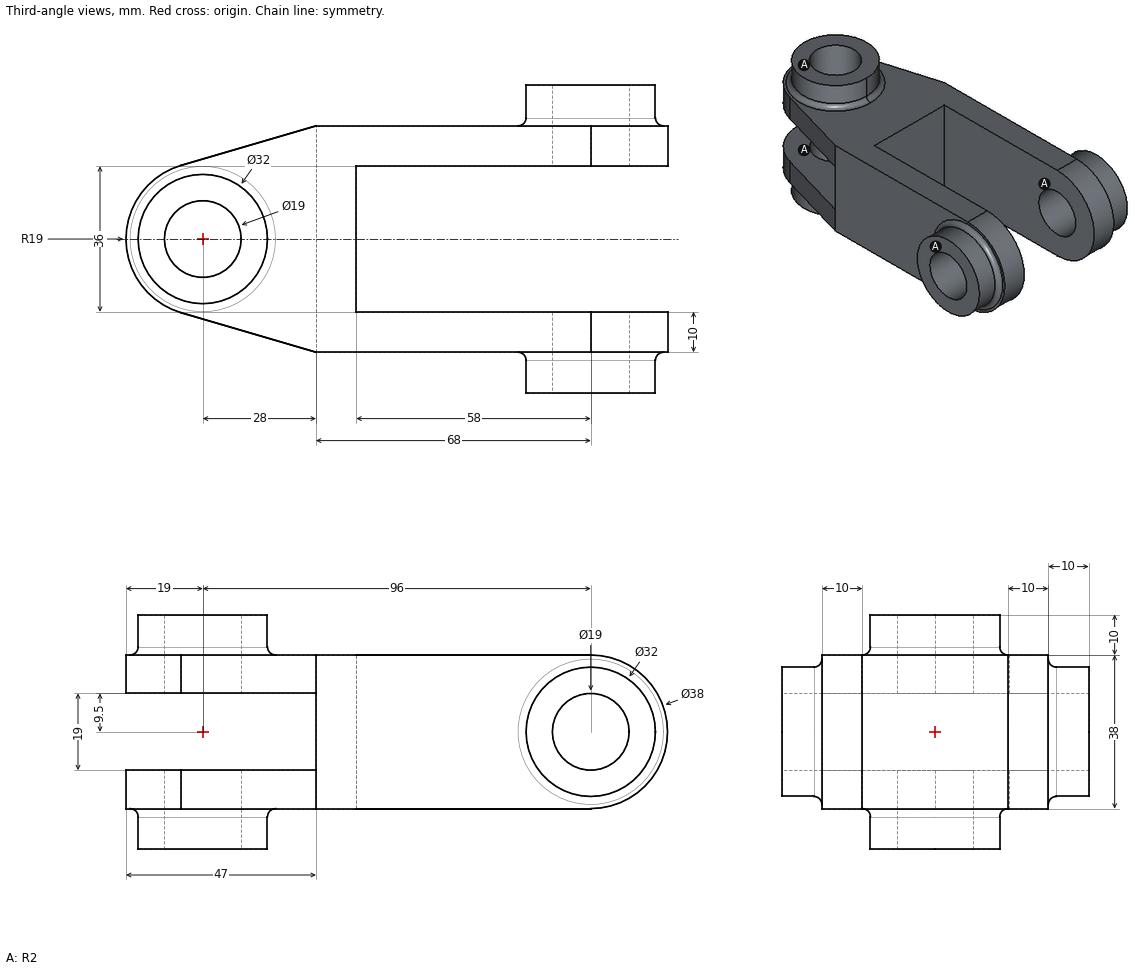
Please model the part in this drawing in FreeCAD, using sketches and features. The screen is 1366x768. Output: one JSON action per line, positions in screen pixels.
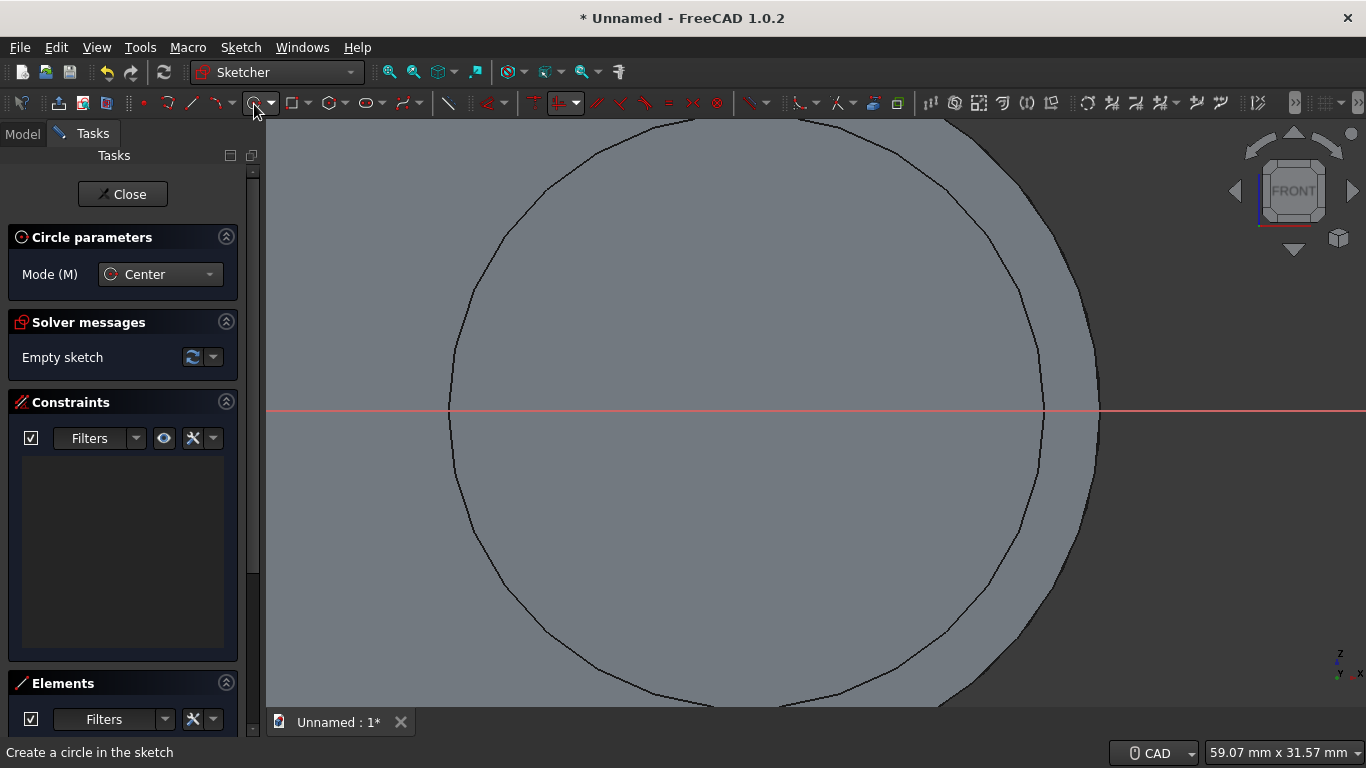
{"action": "left_click", "coordinate": [746, 411]}
{"action": "left_click", "coordinate": [872, 286]}
{"action": "key", "text": "Escape"}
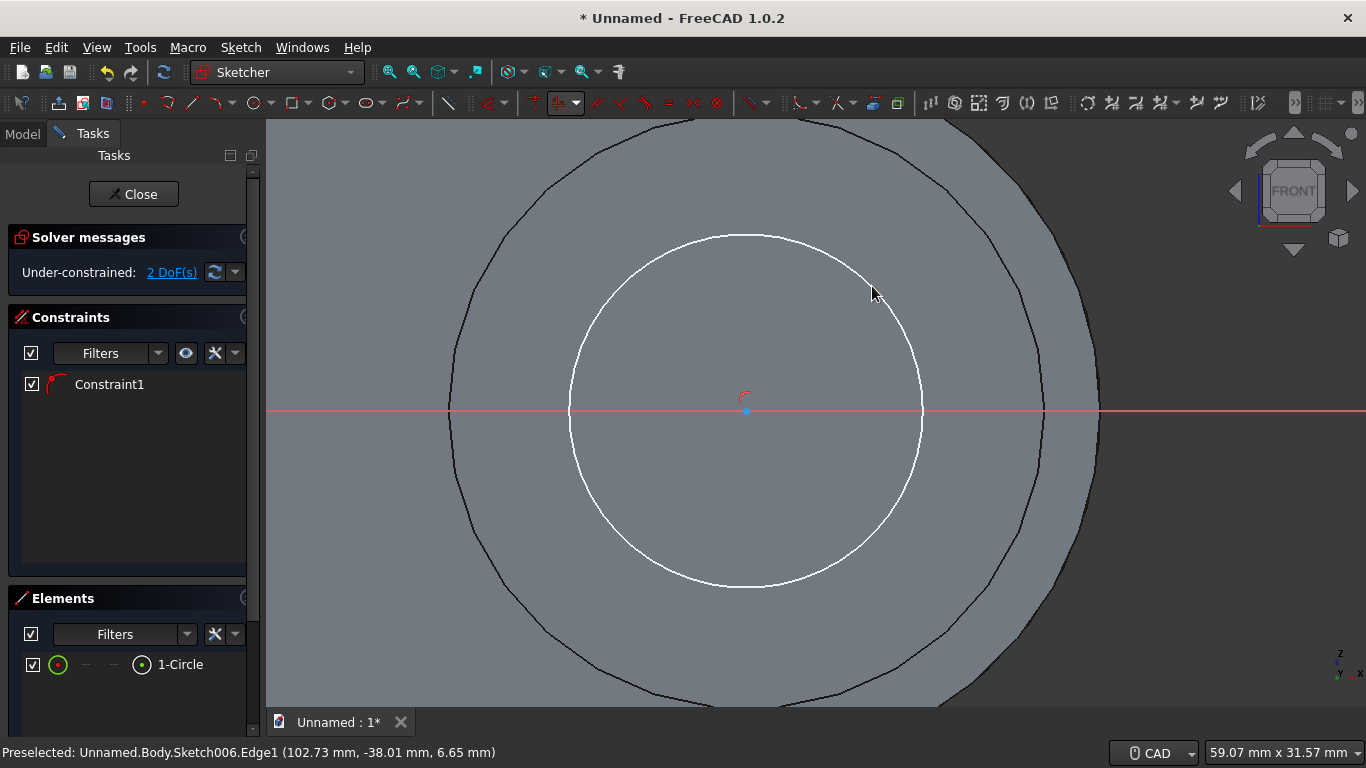
{"action": "left_click", "coordinate": [488, 104]}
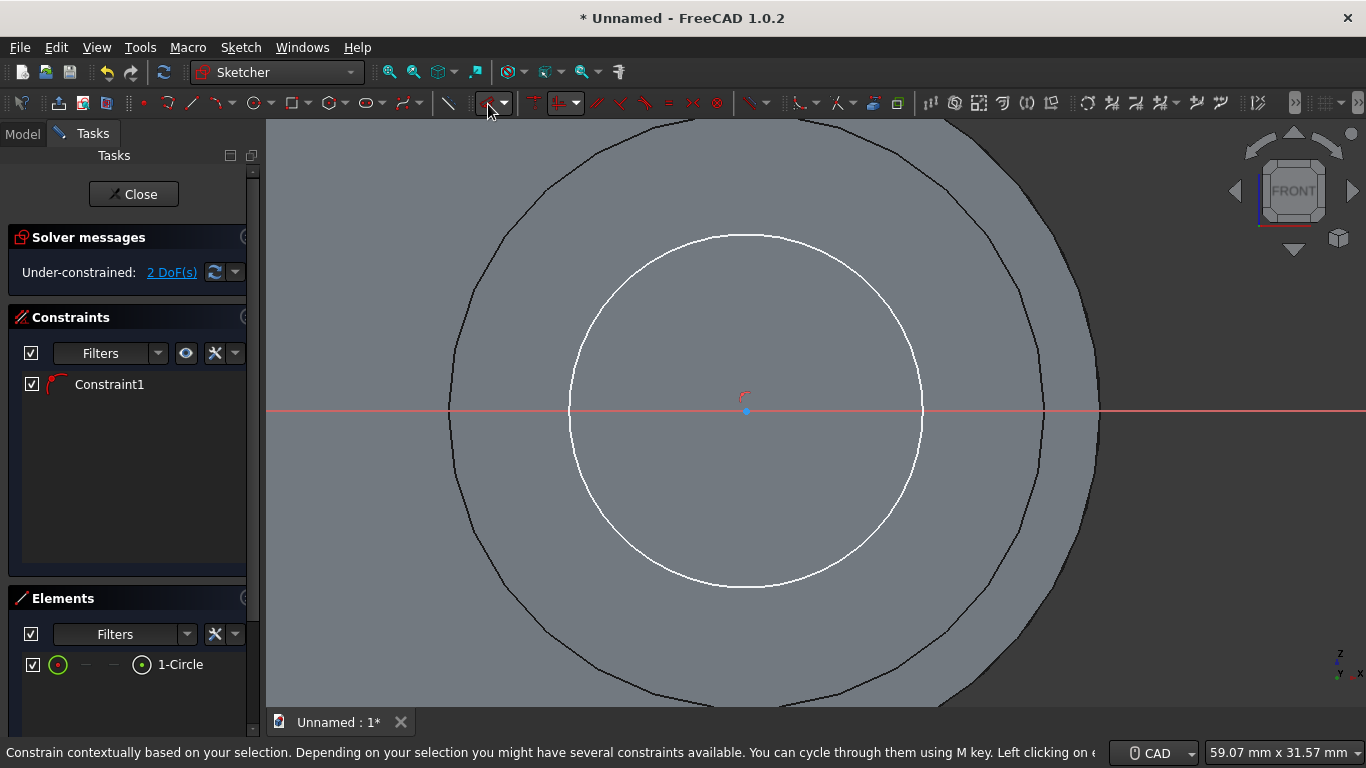
{"action": "left_click", "coordinate": [871, 286]}
{"action": "left_click", "coordinate": [894, 263]}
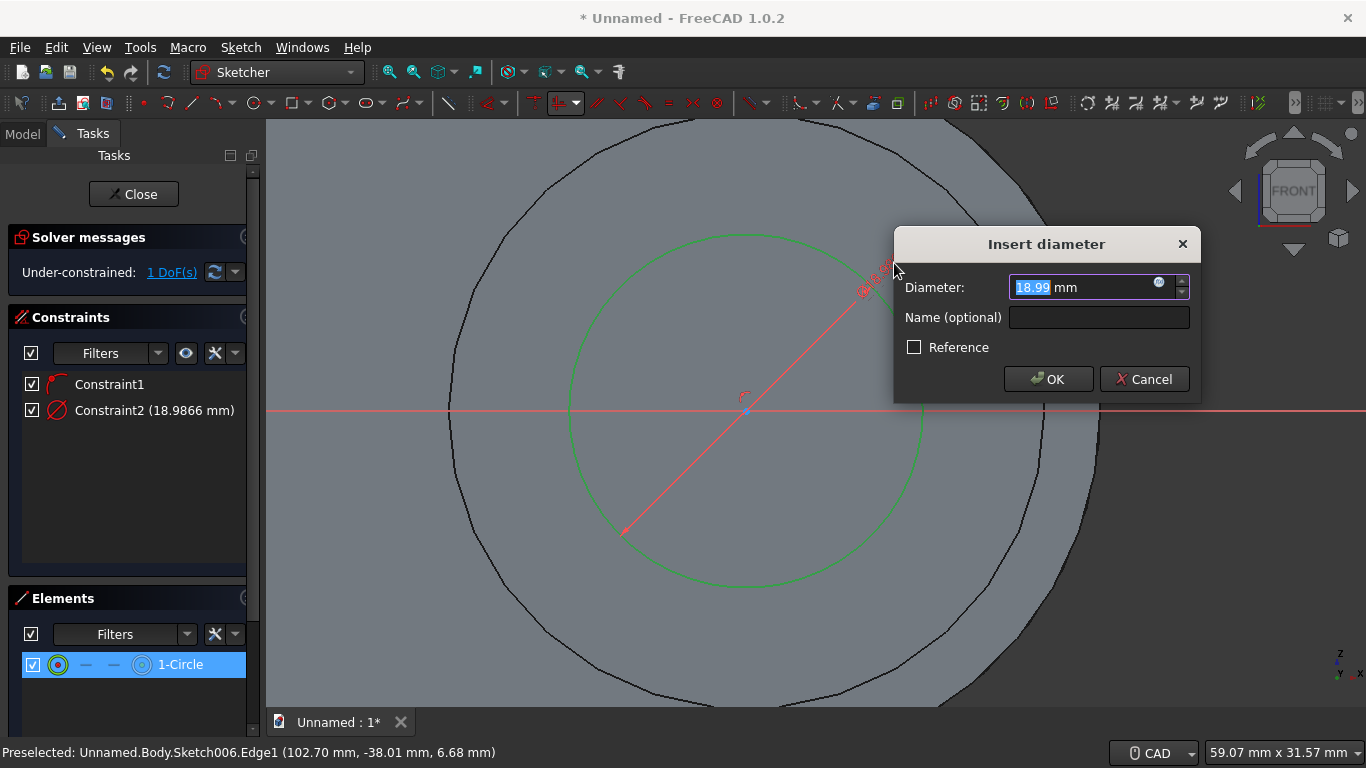
{"action": "type", "text": "19"}
{"action": "key", "text": "Return"}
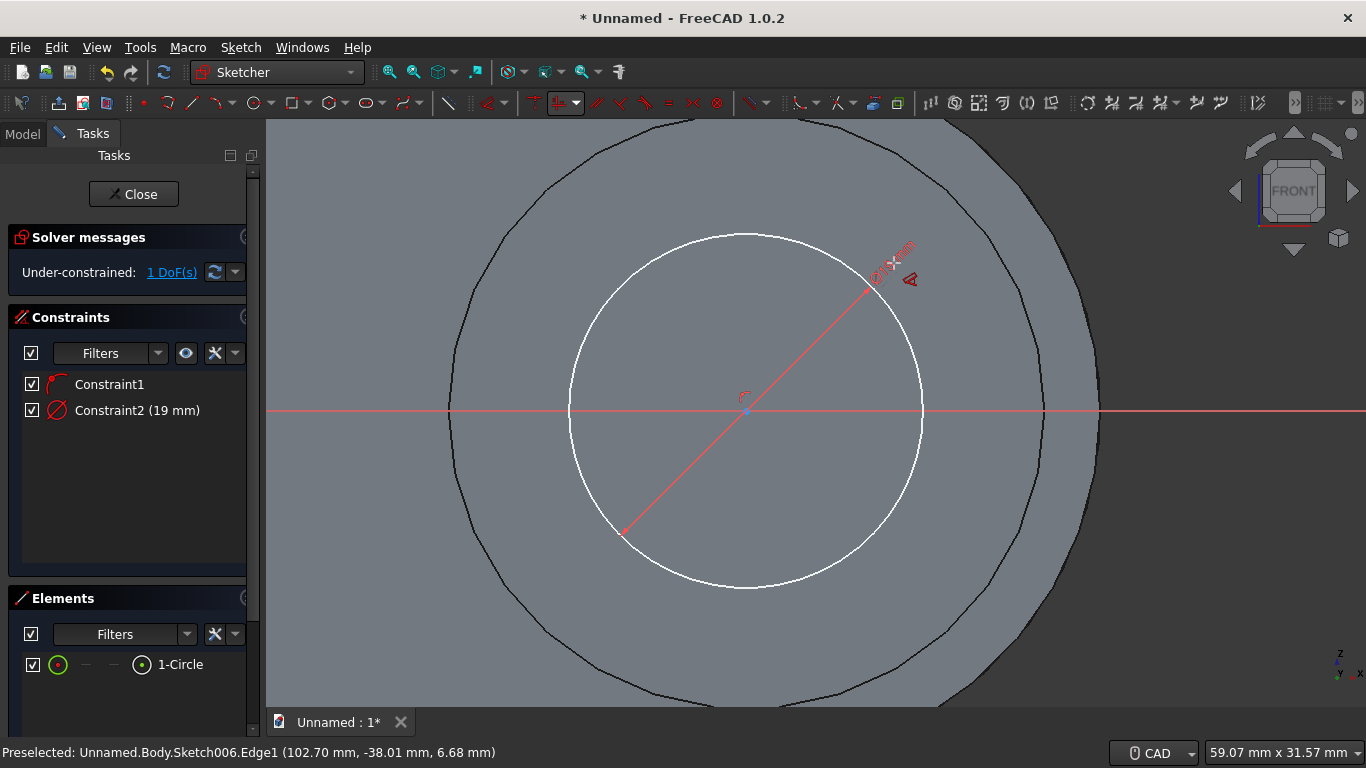
{"action": "left_click", "coordinate": [746, 411]}
{"action": "left_click", "coordinate": [520, 445]}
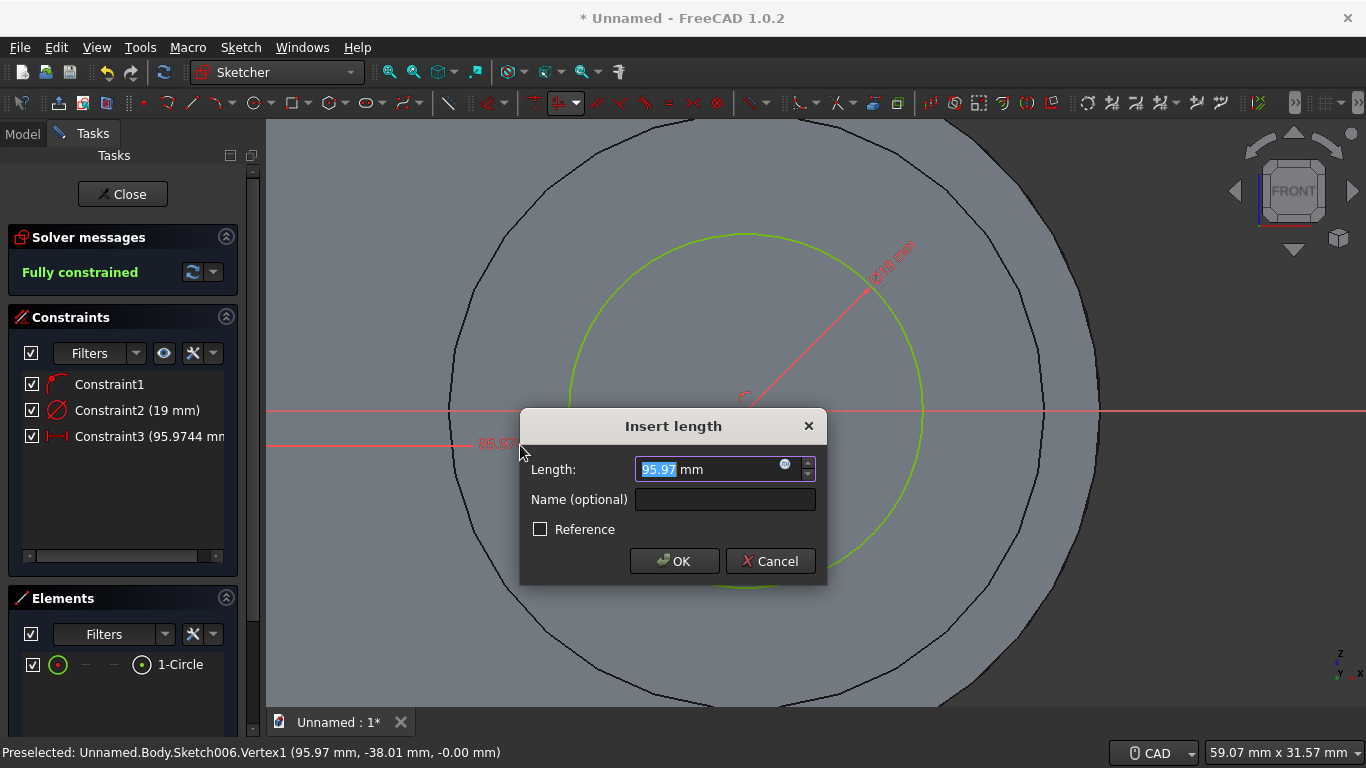
{"action": "type", "text": "96"}
{"action": "key", "text": "Return"}
{"action": "key", "text": "Escape"}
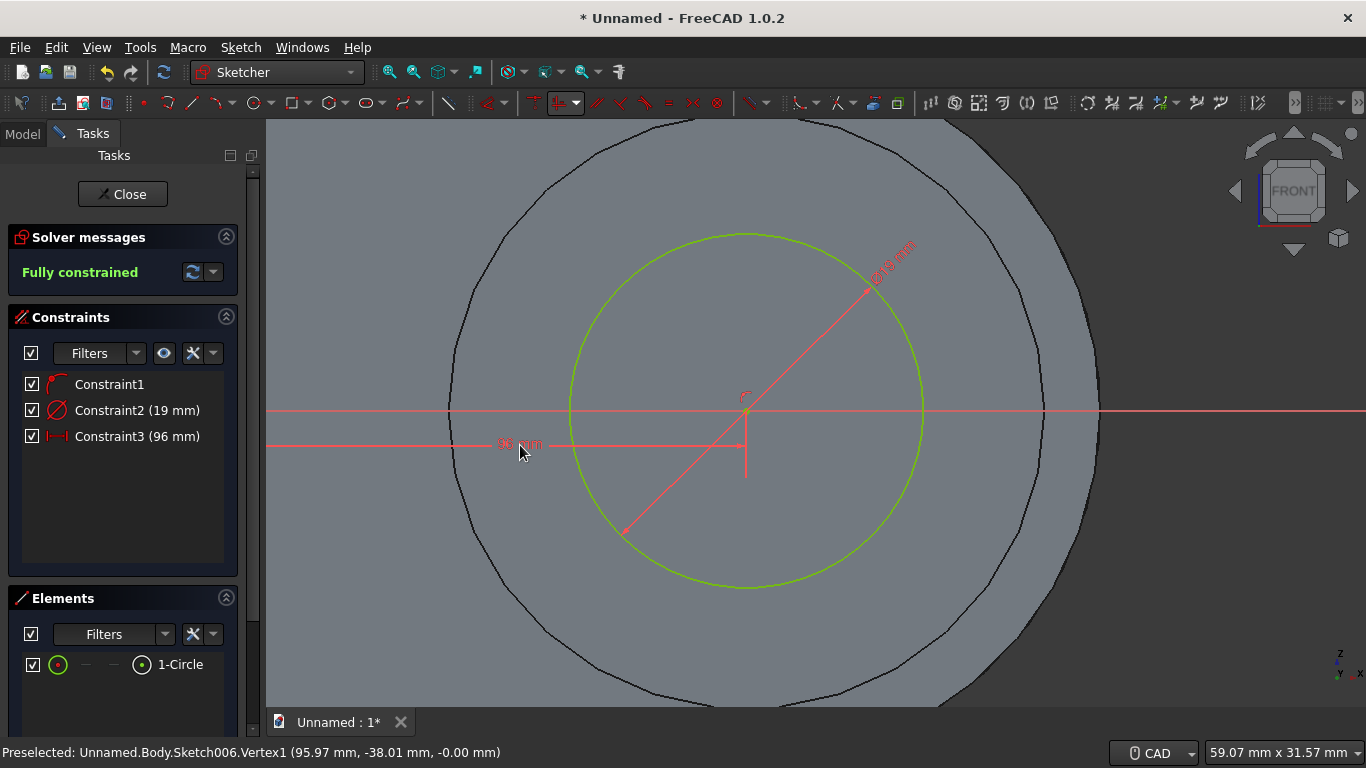
{"action": "left_click", "coordinate": [123, 194]}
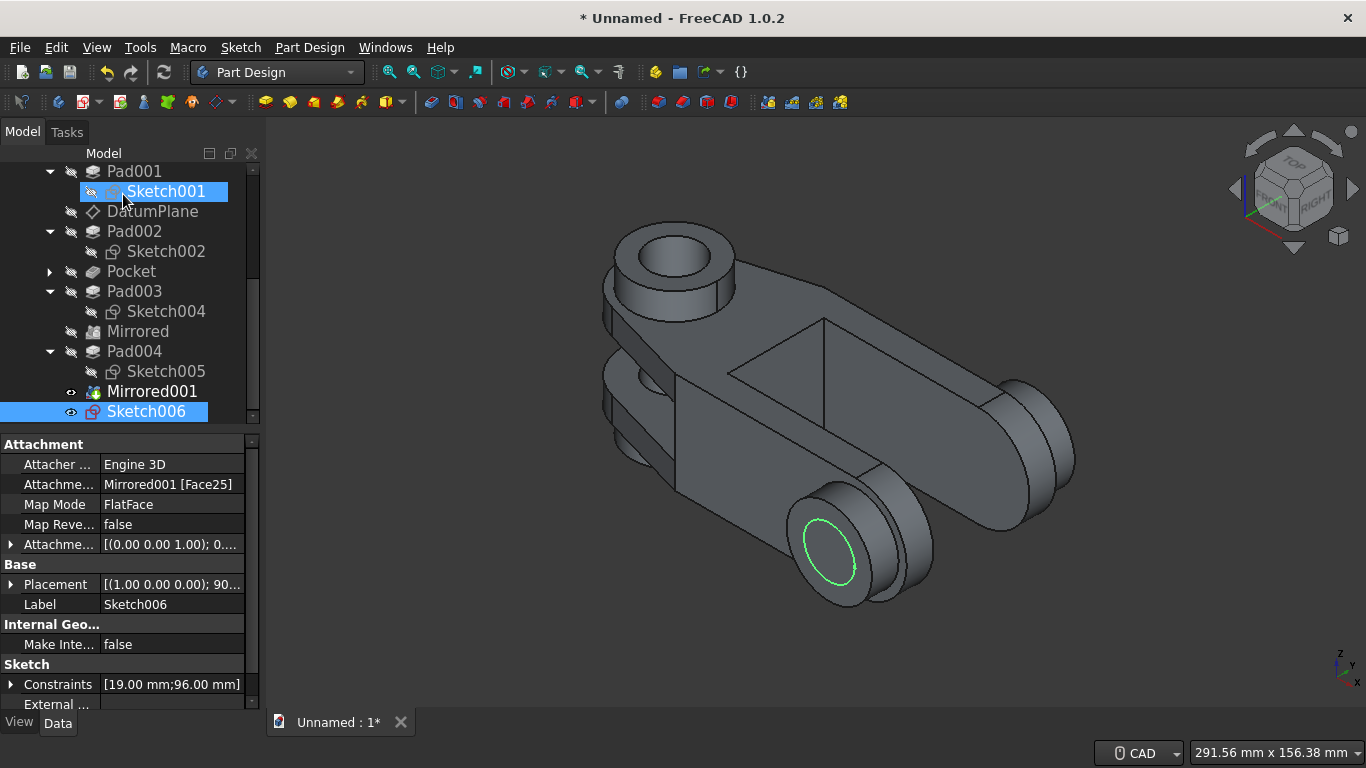
{"action": "left_click", "coordinate": [432, 102]}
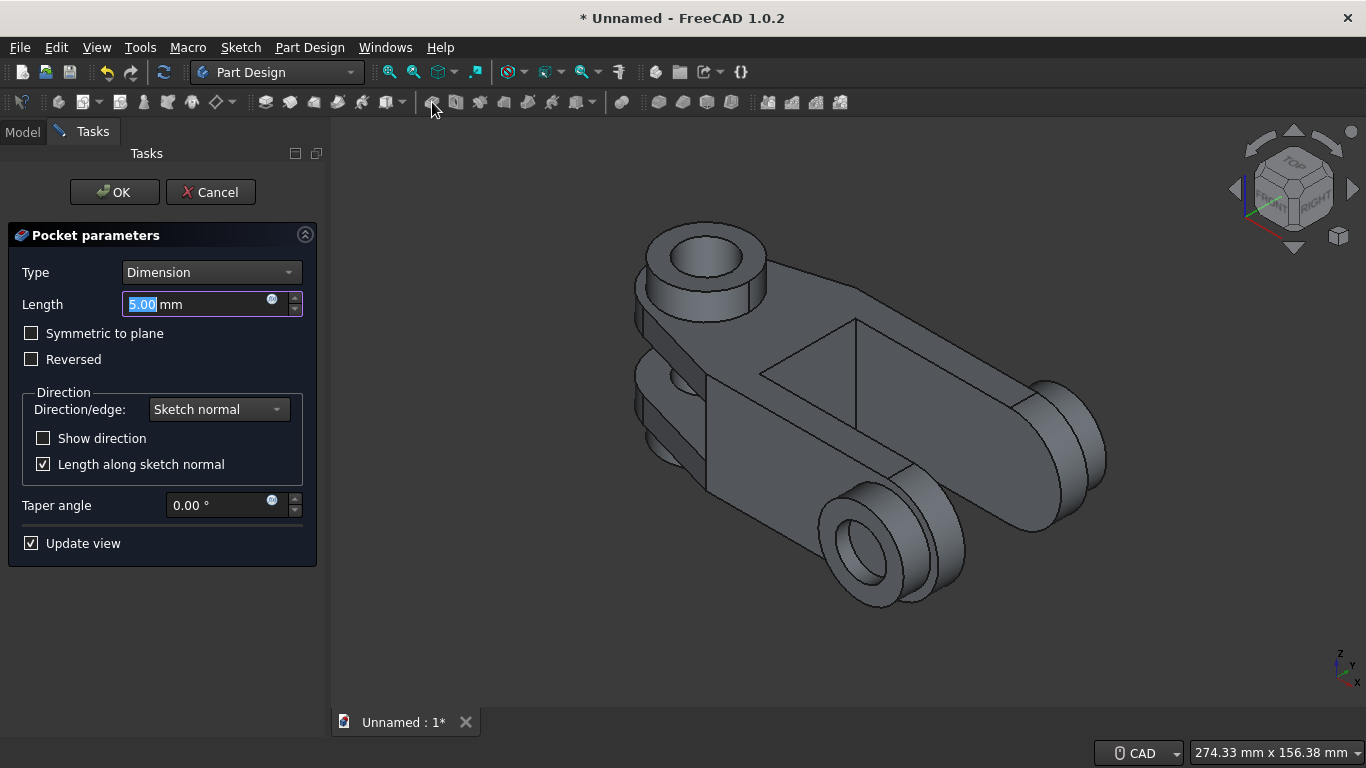
{"action": "left_click", "coordinate": [212, 272]}